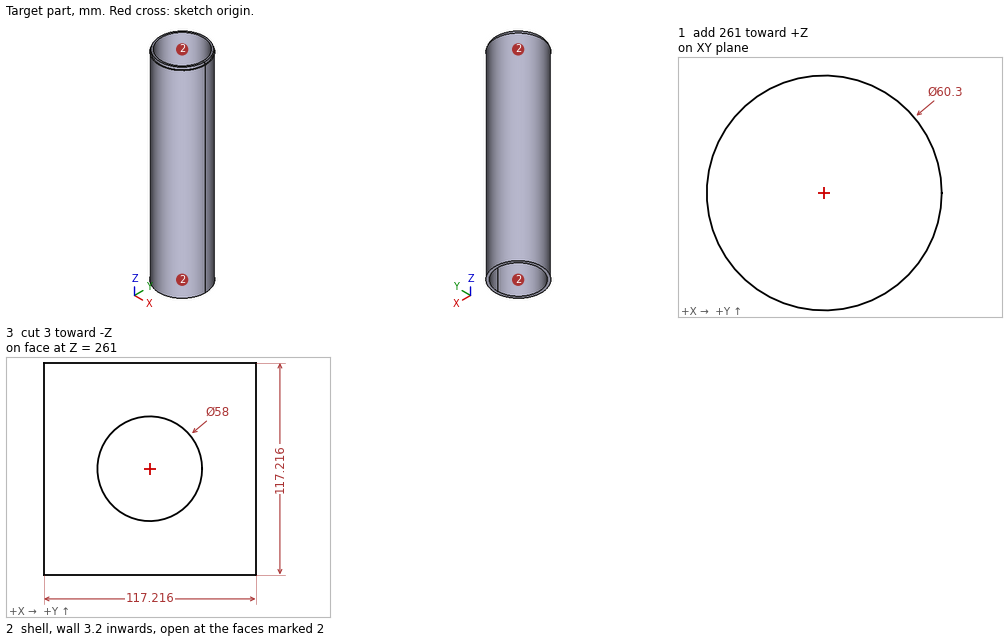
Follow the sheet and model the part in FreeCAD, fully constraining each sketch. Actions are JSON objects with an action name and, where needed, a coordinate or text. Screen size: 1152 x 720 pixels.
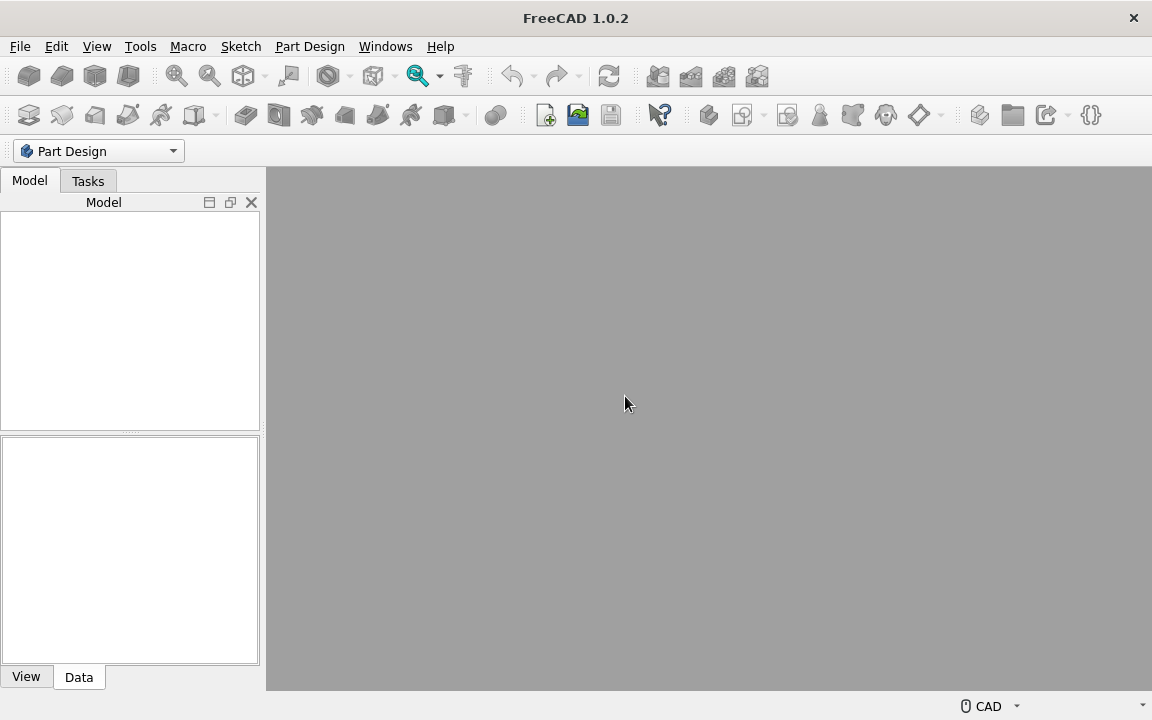
{"action": "key", "text": "ctrl+n"}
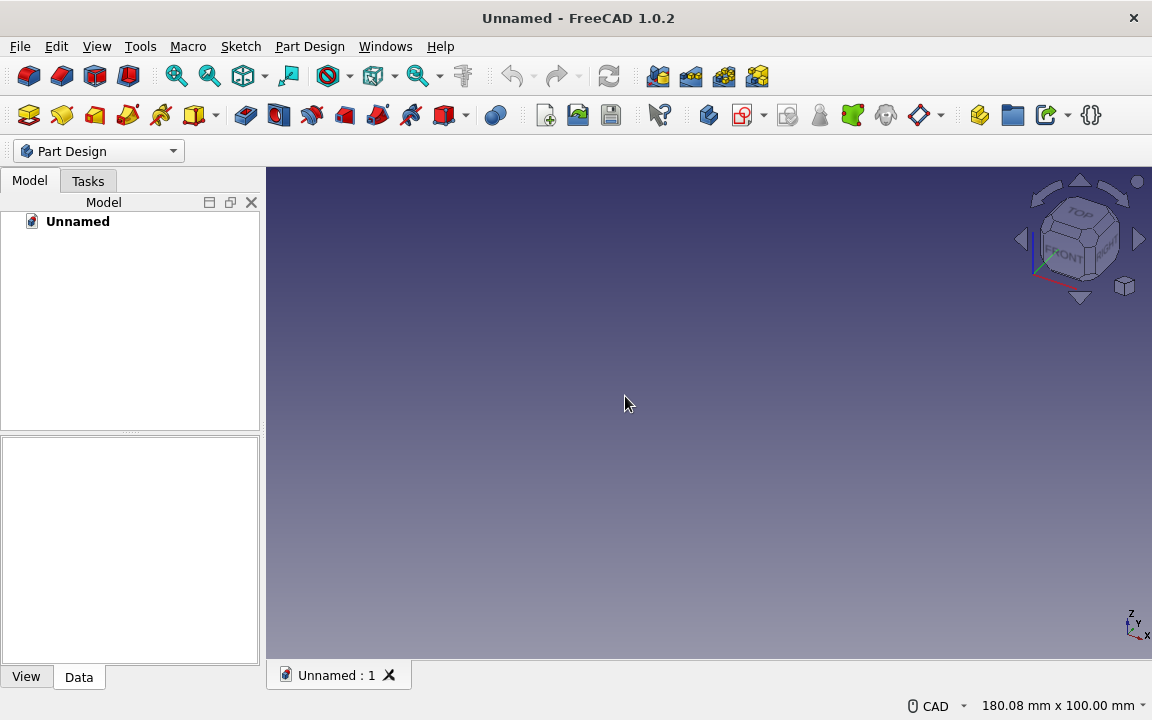
{"action": "left_click", "coordinate": [742, 116]}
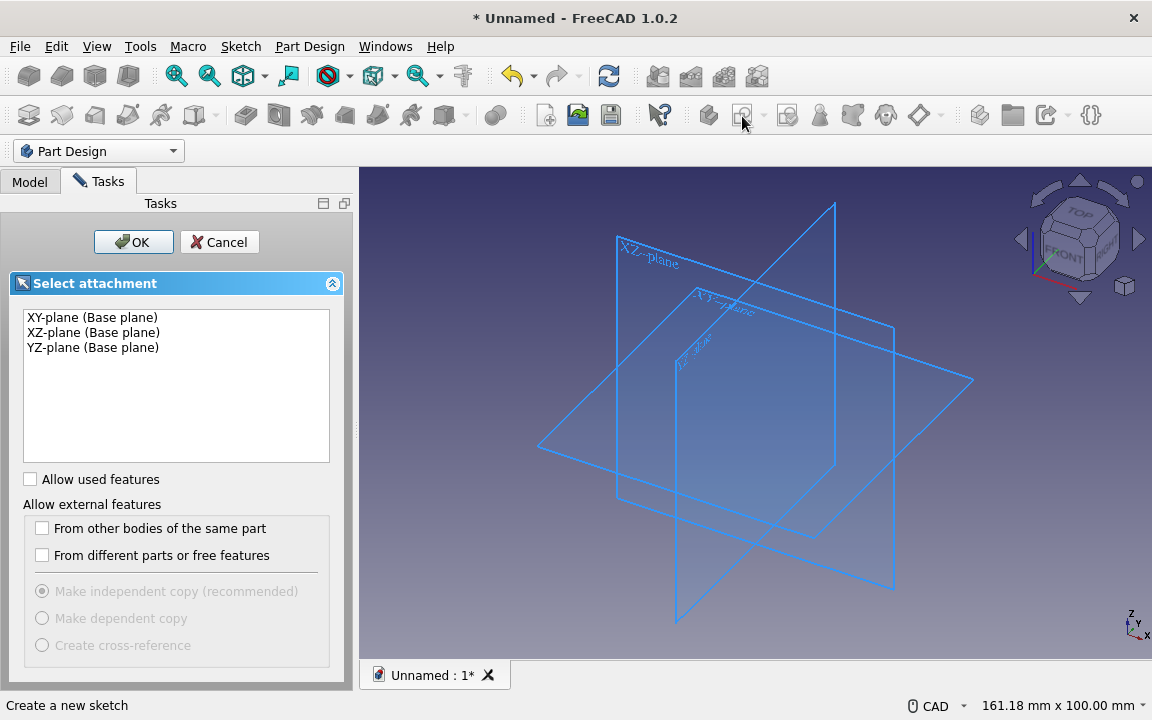
{"action": "left_click", "coordinate": [84, 318]}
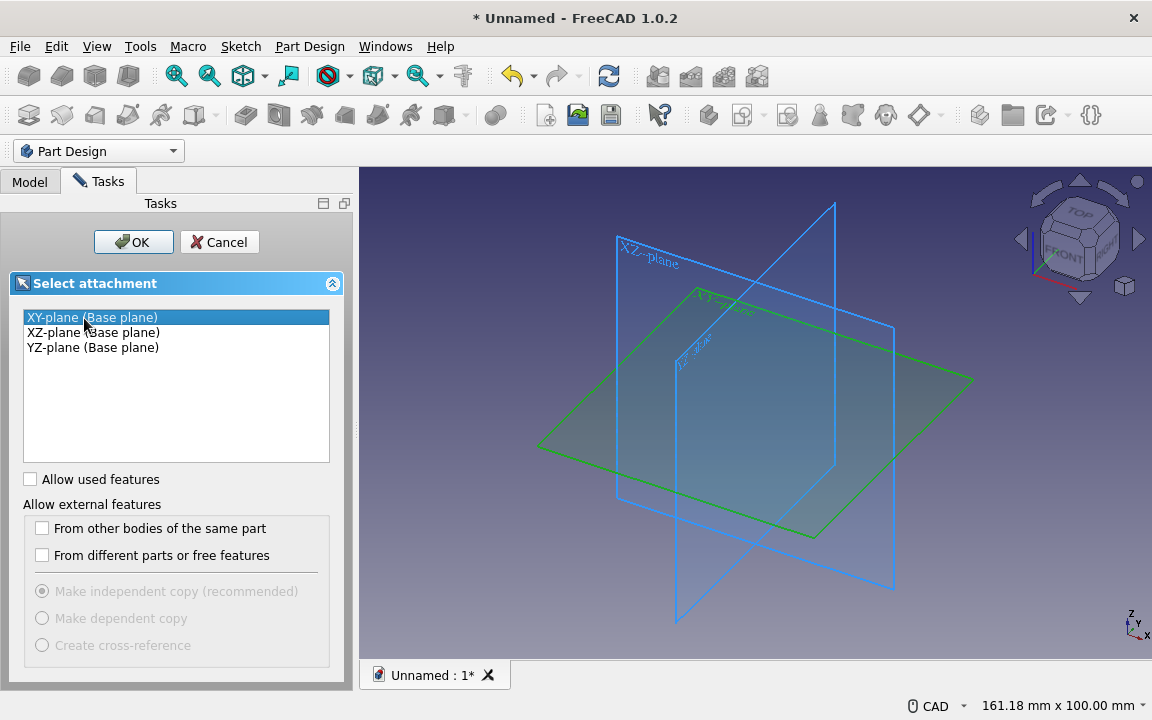
{"action": "left_click", "coordinate": [134, 242]}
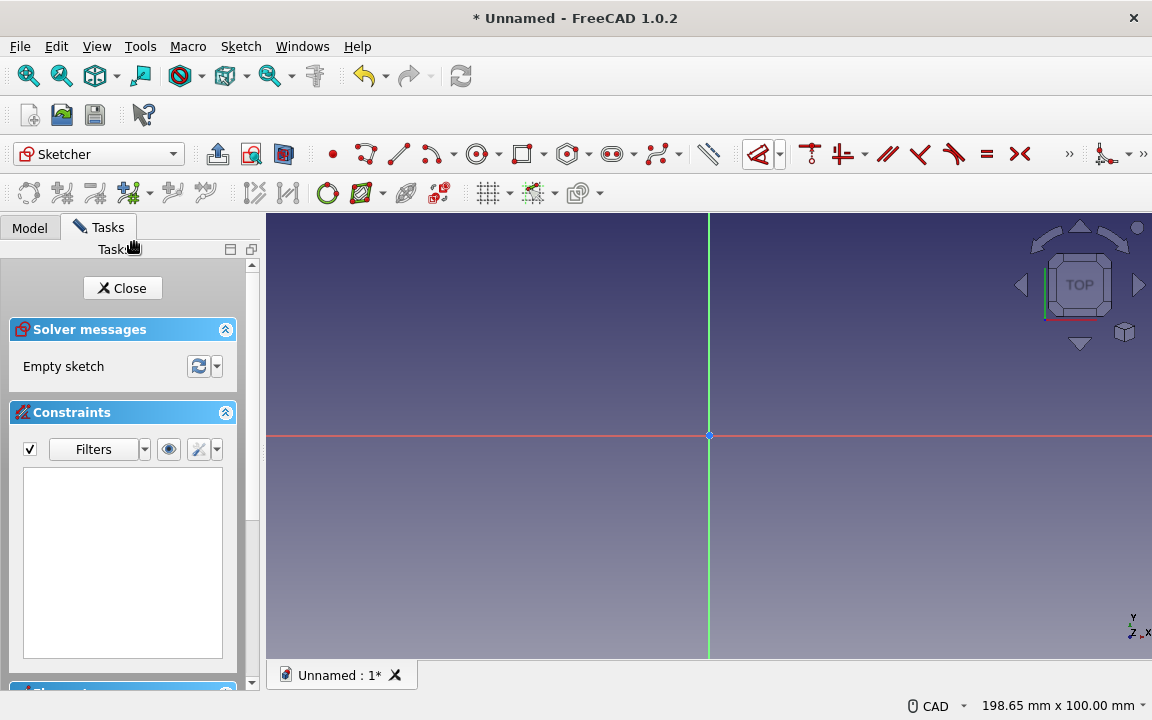
{"action": "key", "text": "g c"}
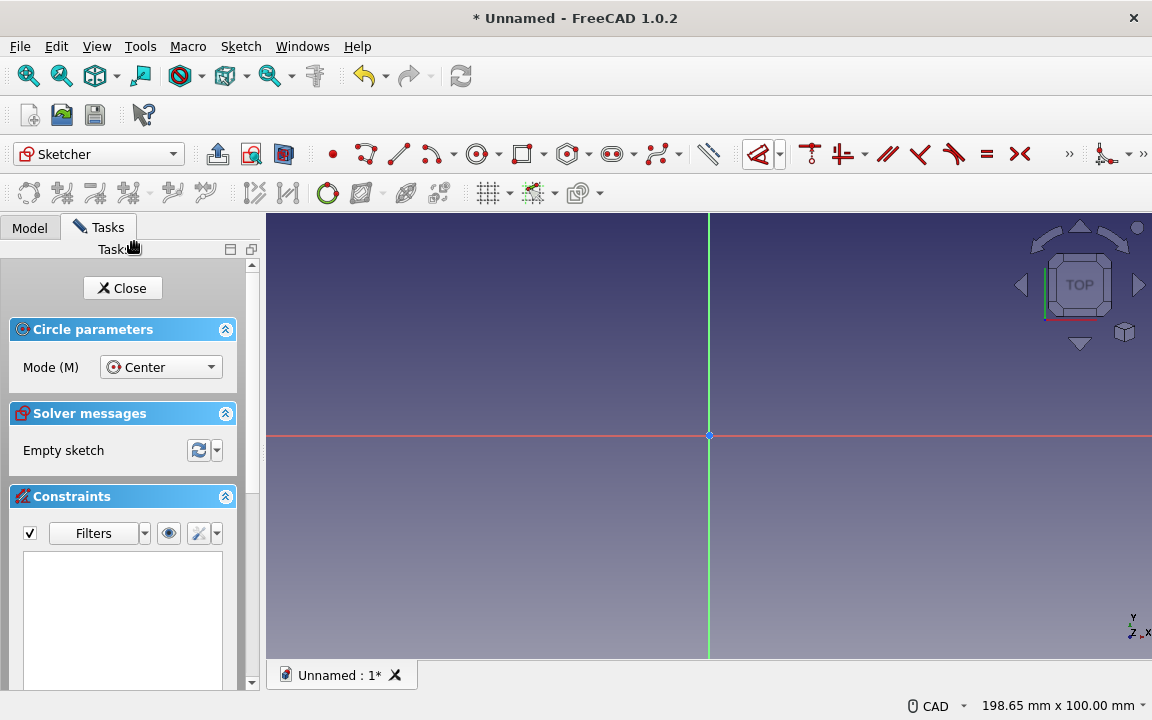
{"action": "left_click", "coordinate": [709, 436]}
{"action": "mouse_move", "coordinate": [804, 341]}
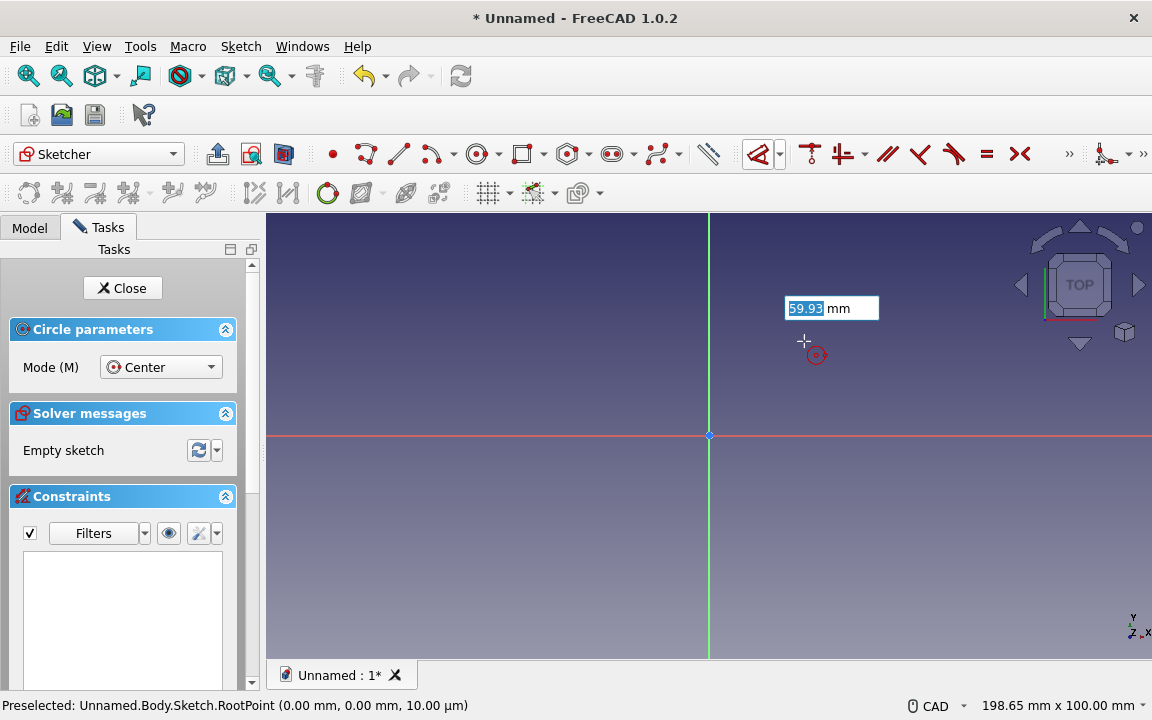
{"action": "type", "text": "60.3"}
{"action": "key", "text": "Return"}
{"action": "key", "text": "Escape"}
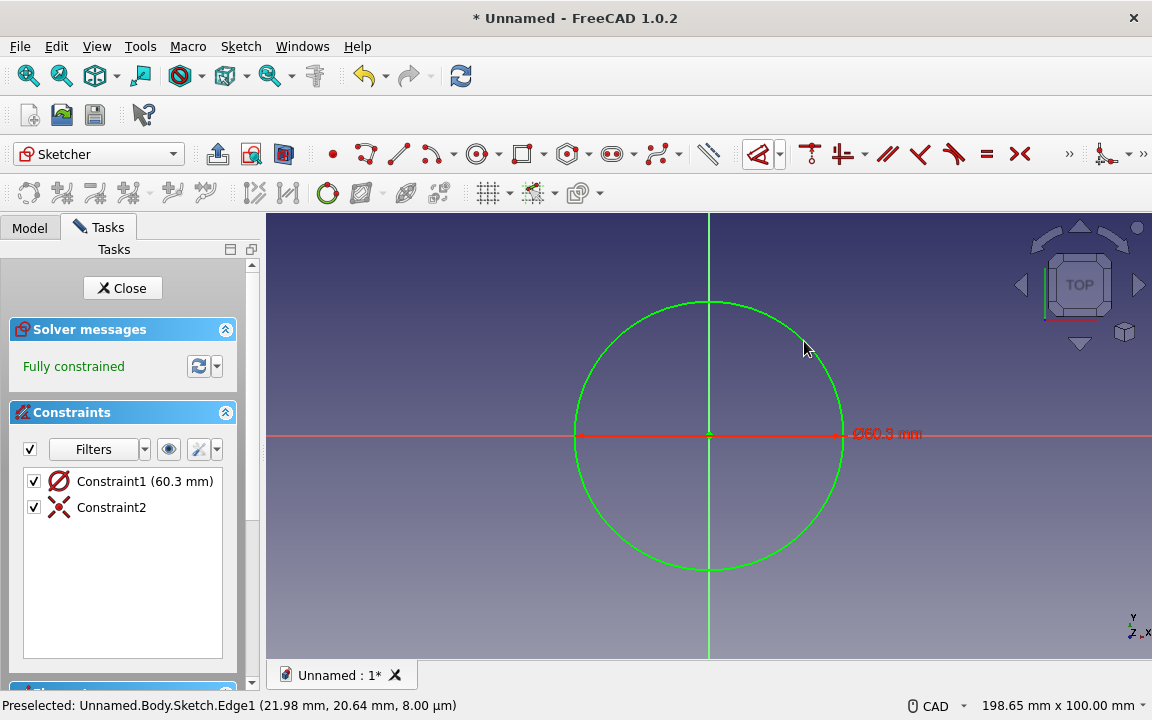
{"action": "left_click", "coordinate": [123, 288]}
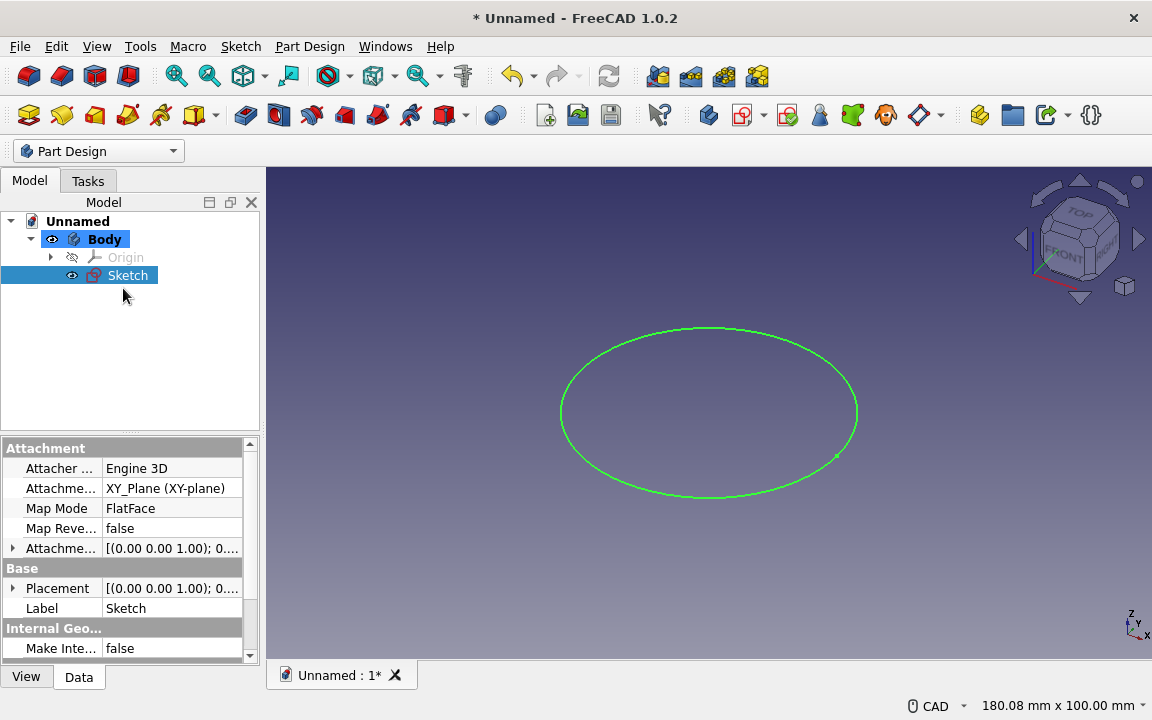
{"action": "left_click", "coordinate": [29, 116]}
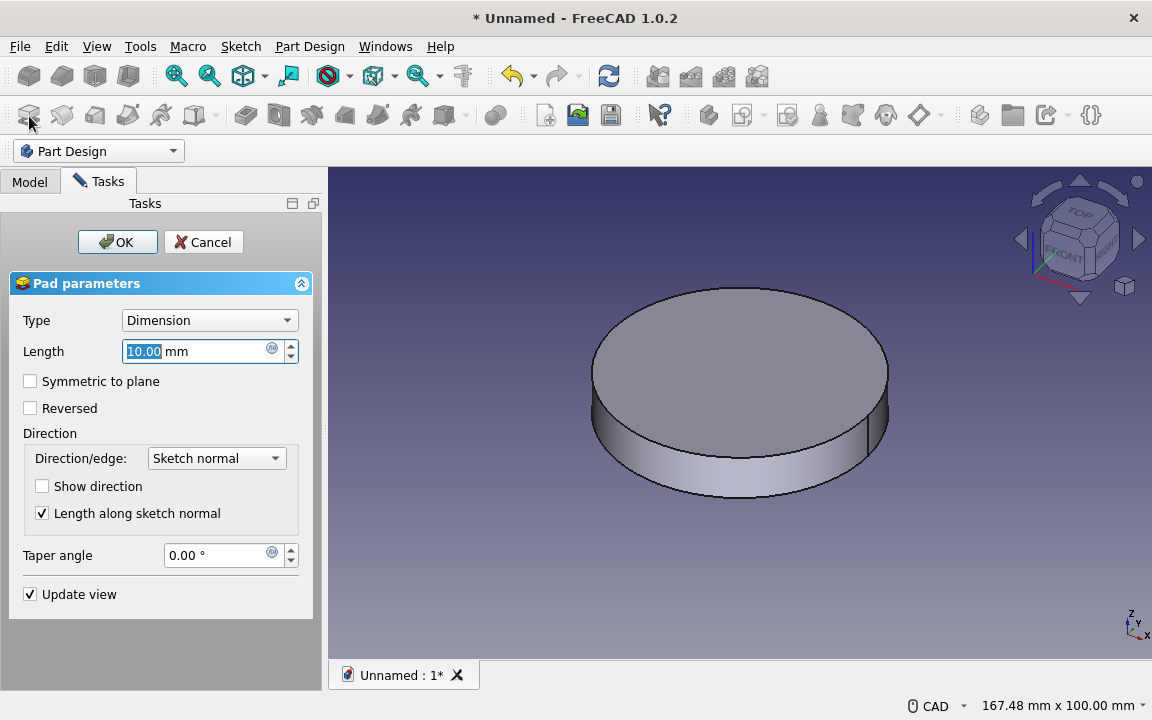
{"action": "type", "text": "261"}
{"action": "key", "text": "Tab"}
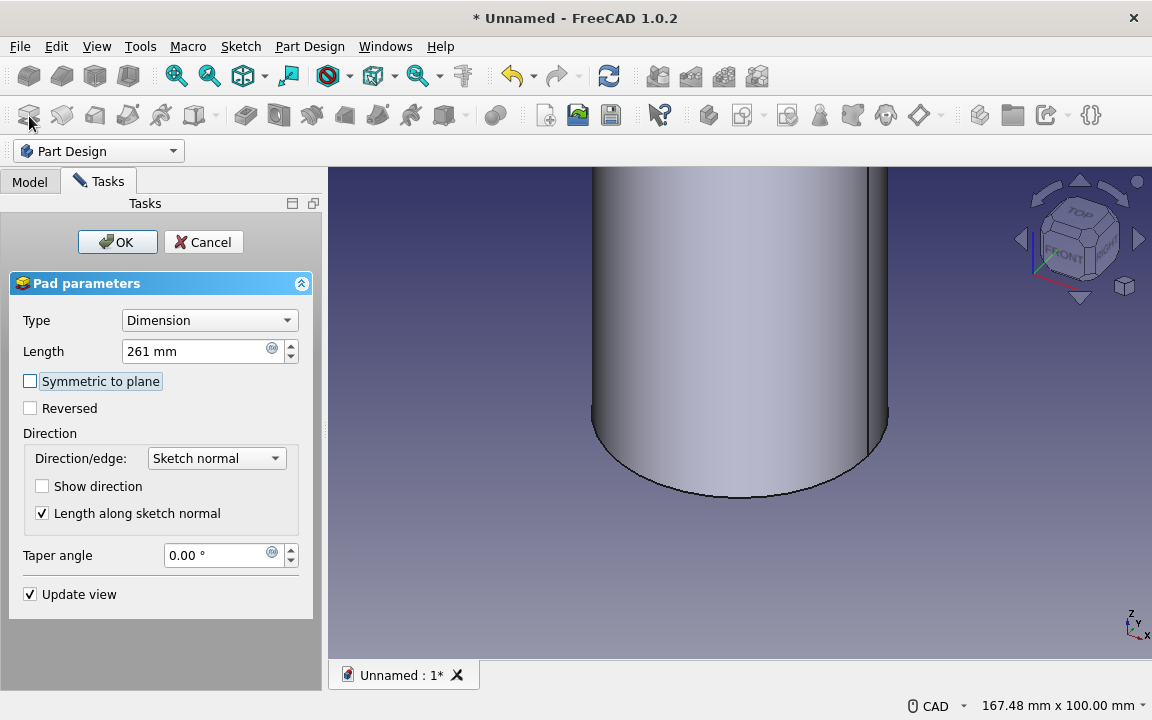
{"action": "left_click", "coordinate": [118, 242]}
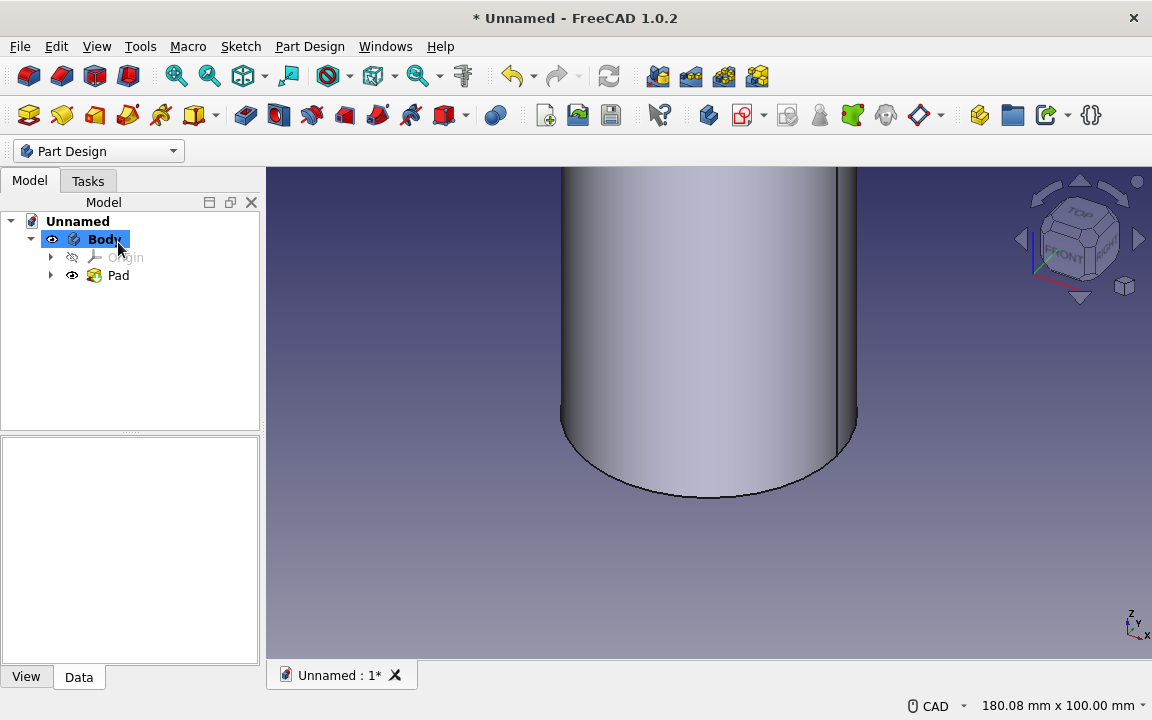
{"action": "key", "text": "v f"}